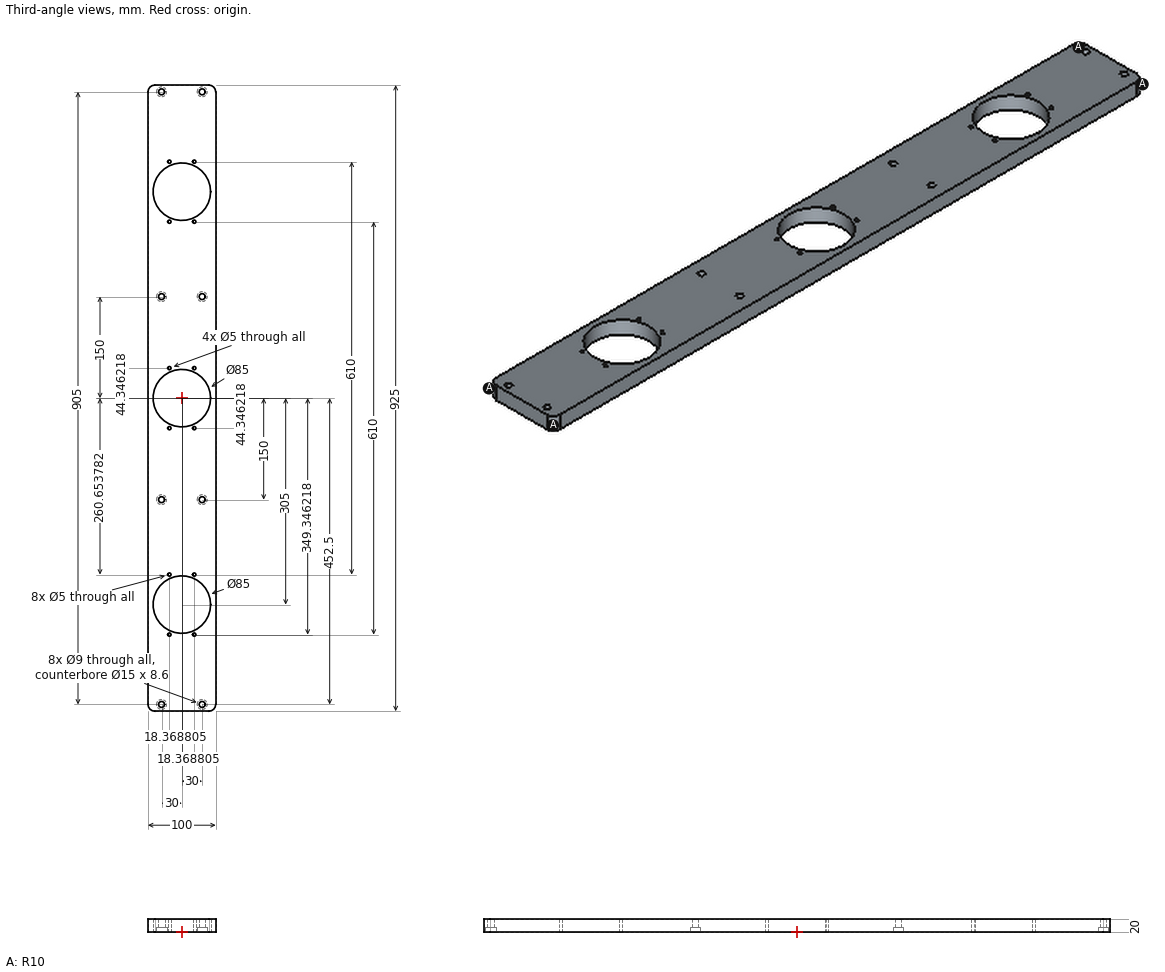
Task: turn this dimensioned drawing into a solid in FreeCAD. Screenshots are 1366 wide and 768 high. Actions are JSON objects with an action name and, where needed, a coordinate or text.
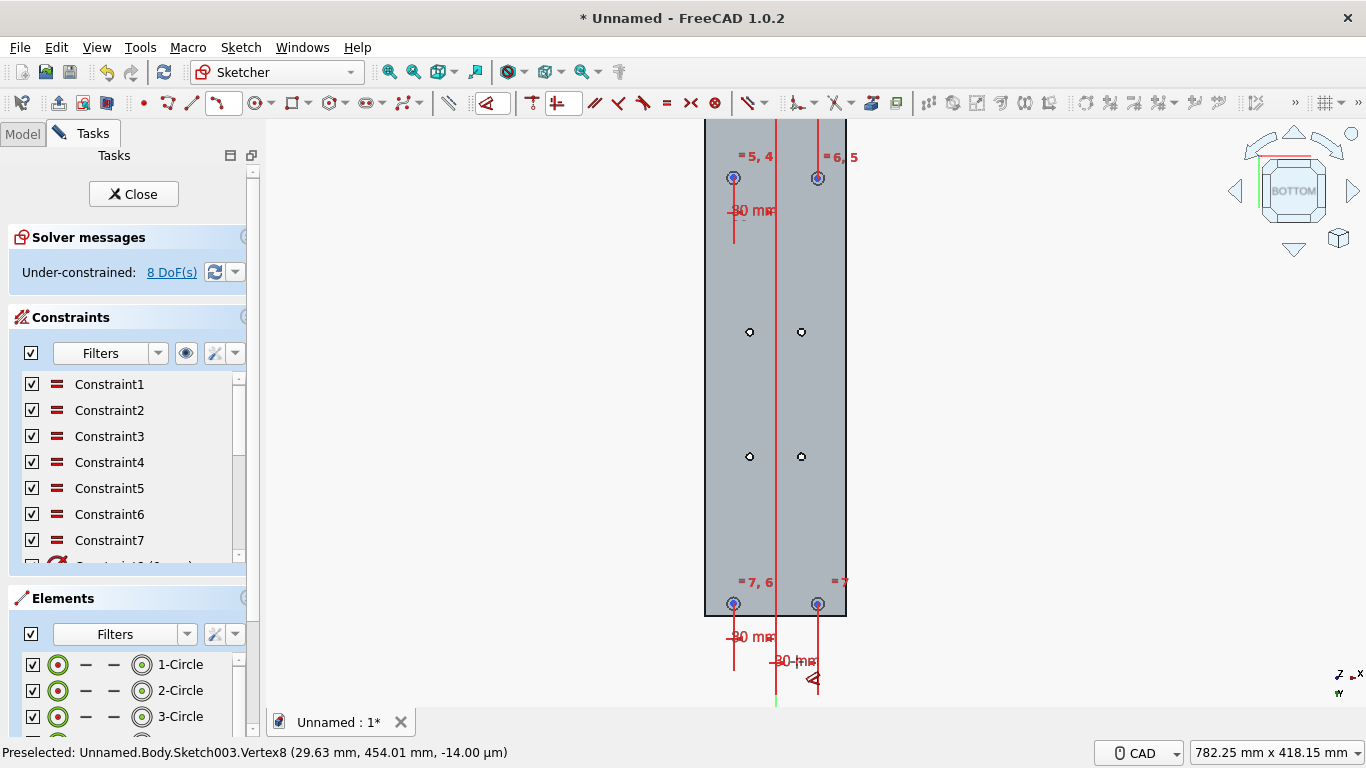
{"action": "scroll", "coordinate": [735, 606], "scroll_direction": "down", "scroll_amount": 6}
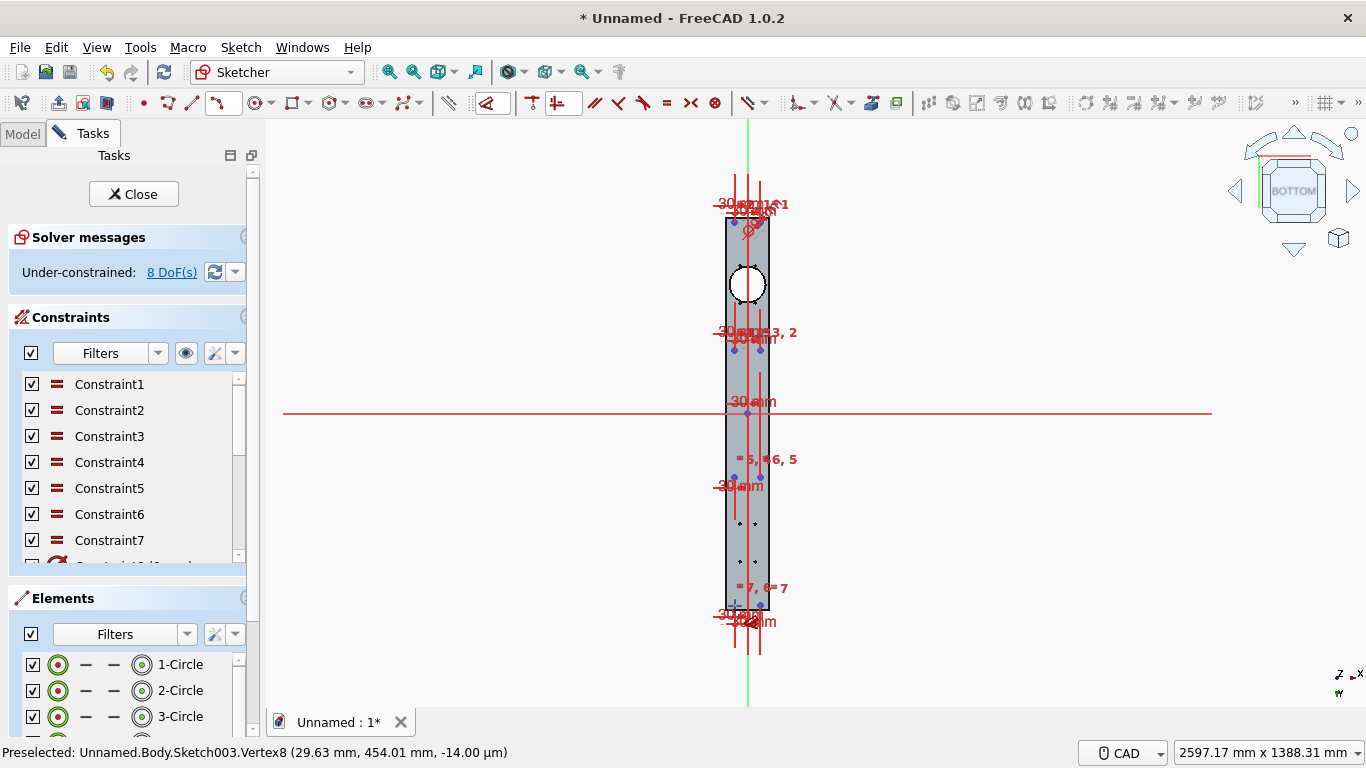
{"action": "left_click", "coordinate": [760, 351]}
{"action": "left_click", "coordinate": [794, 382]}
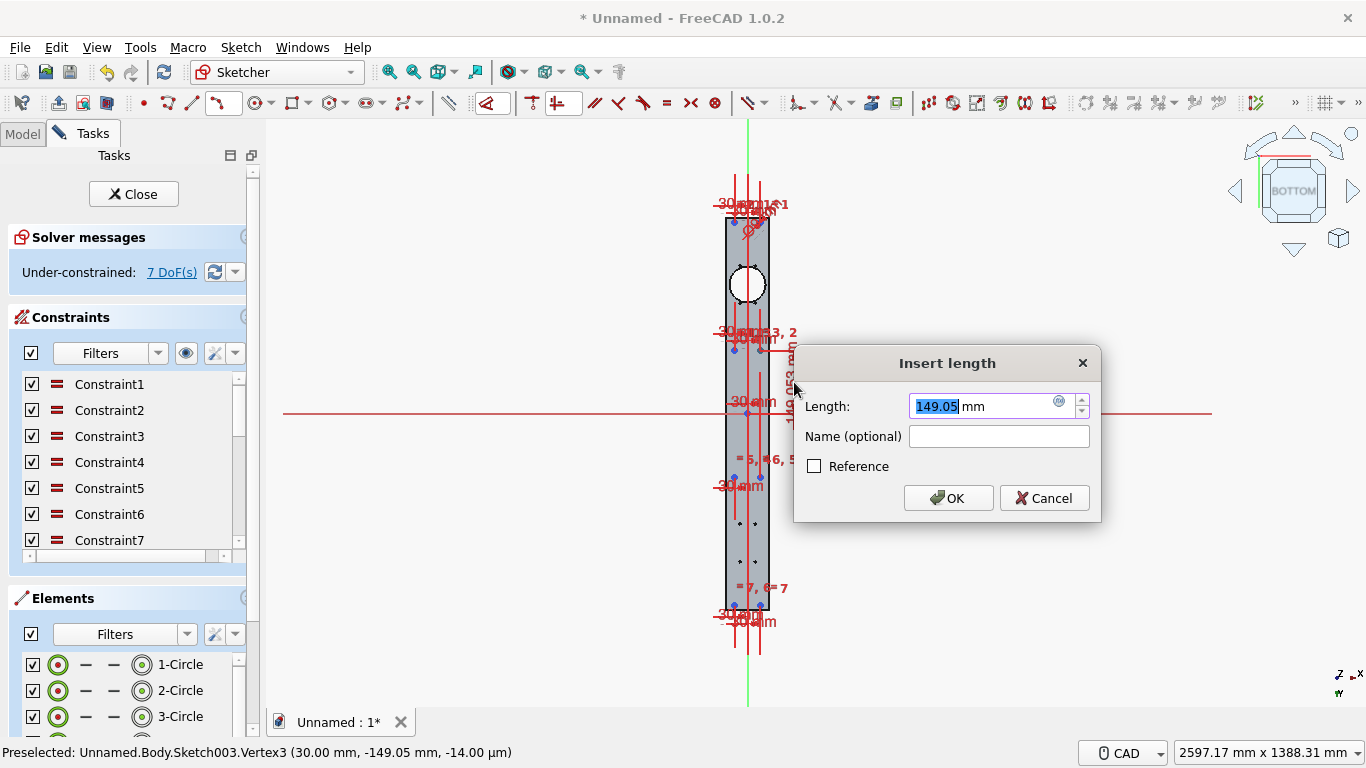
{"action": "type", "text": "150"}
{"action": "key", "text": "Return"}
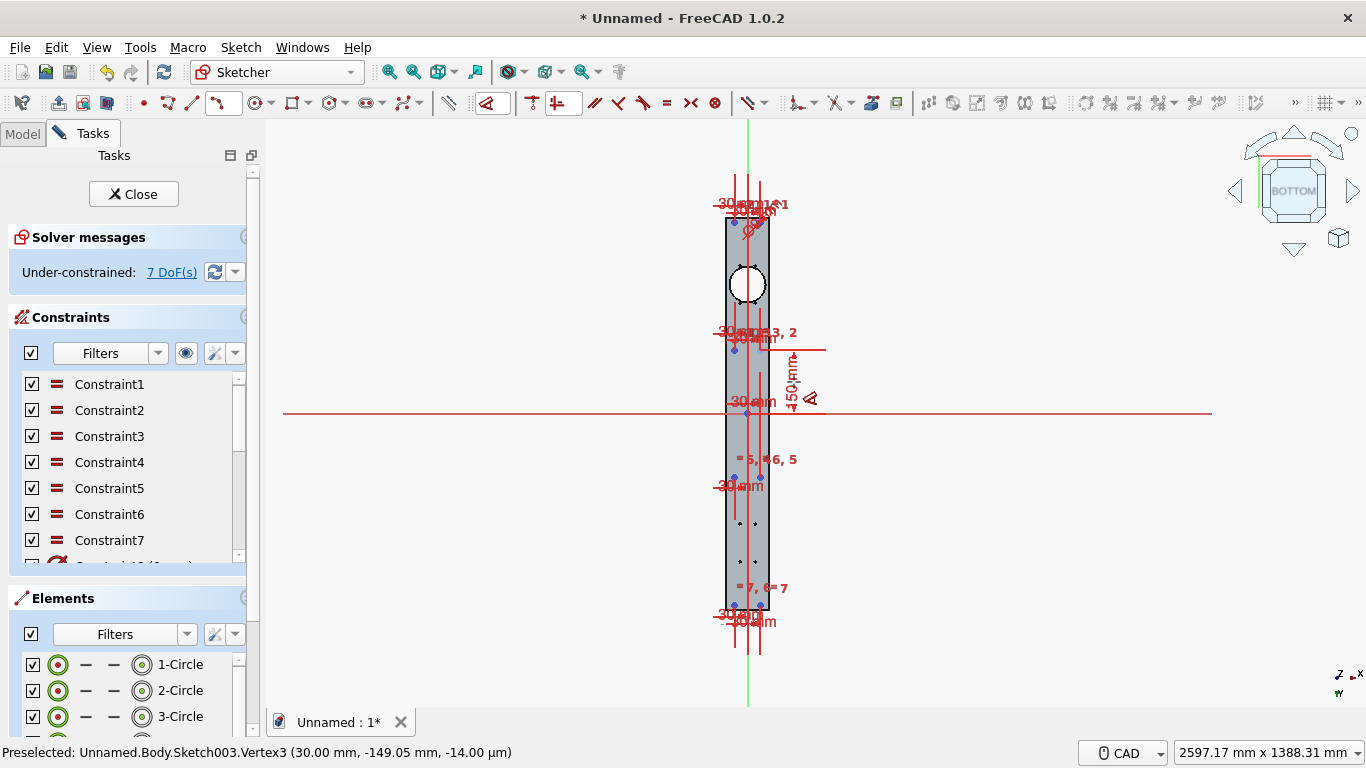
{"action": "left_click", "coordinate": [735, 351]}
{"action": "left_click", "coordinate": [701, 382]}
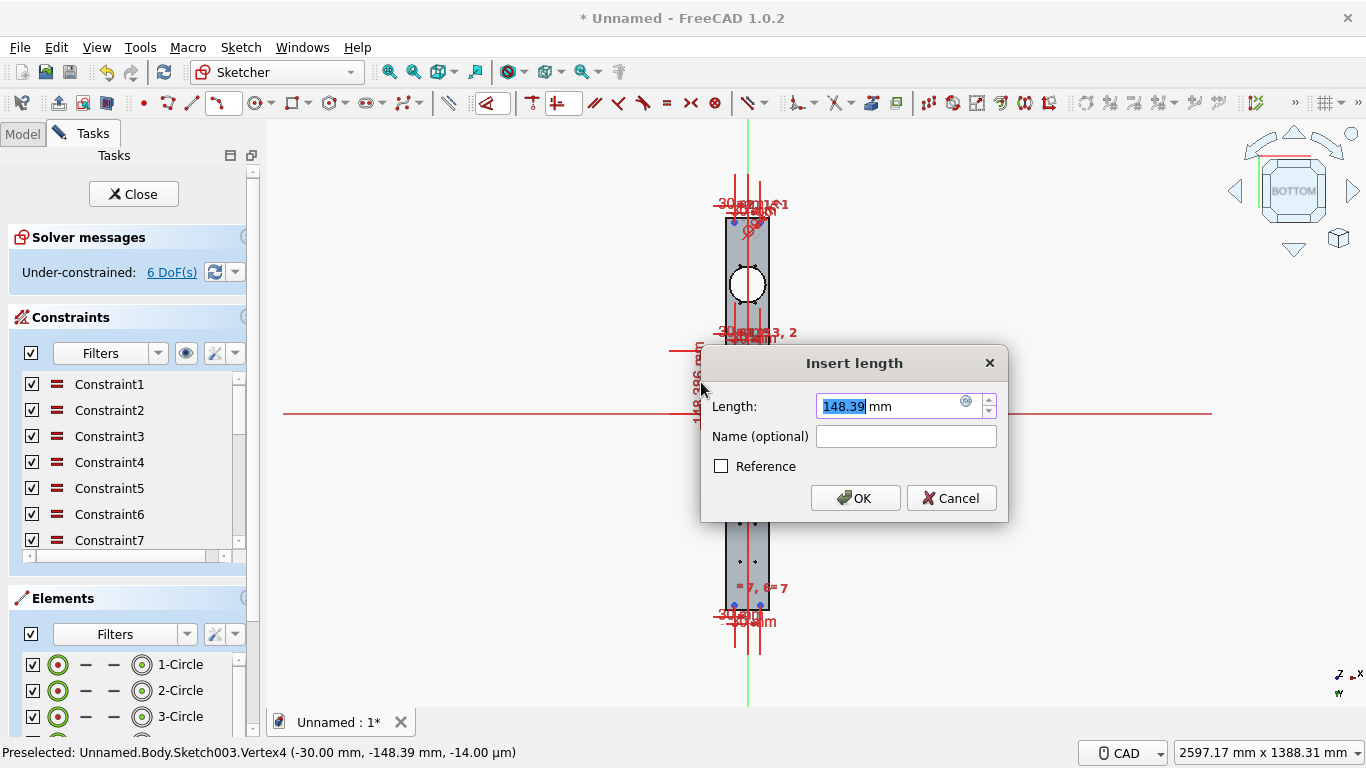
{"action": "type", "text": "150"}
{"action": "key", "text": "Return"}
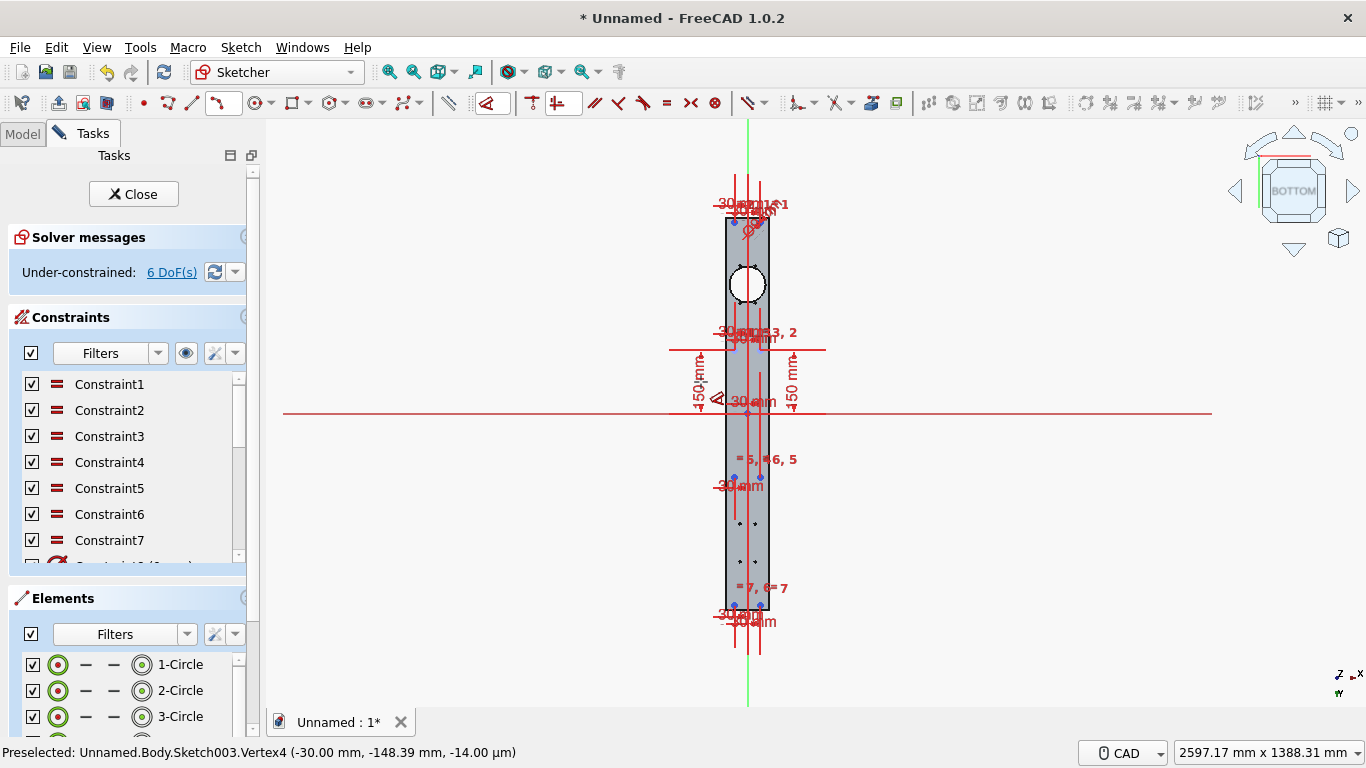
{"action": "left_click", "coordinate": [735, 478]}
{"action": "left_click", "coordinate": [701, 446]}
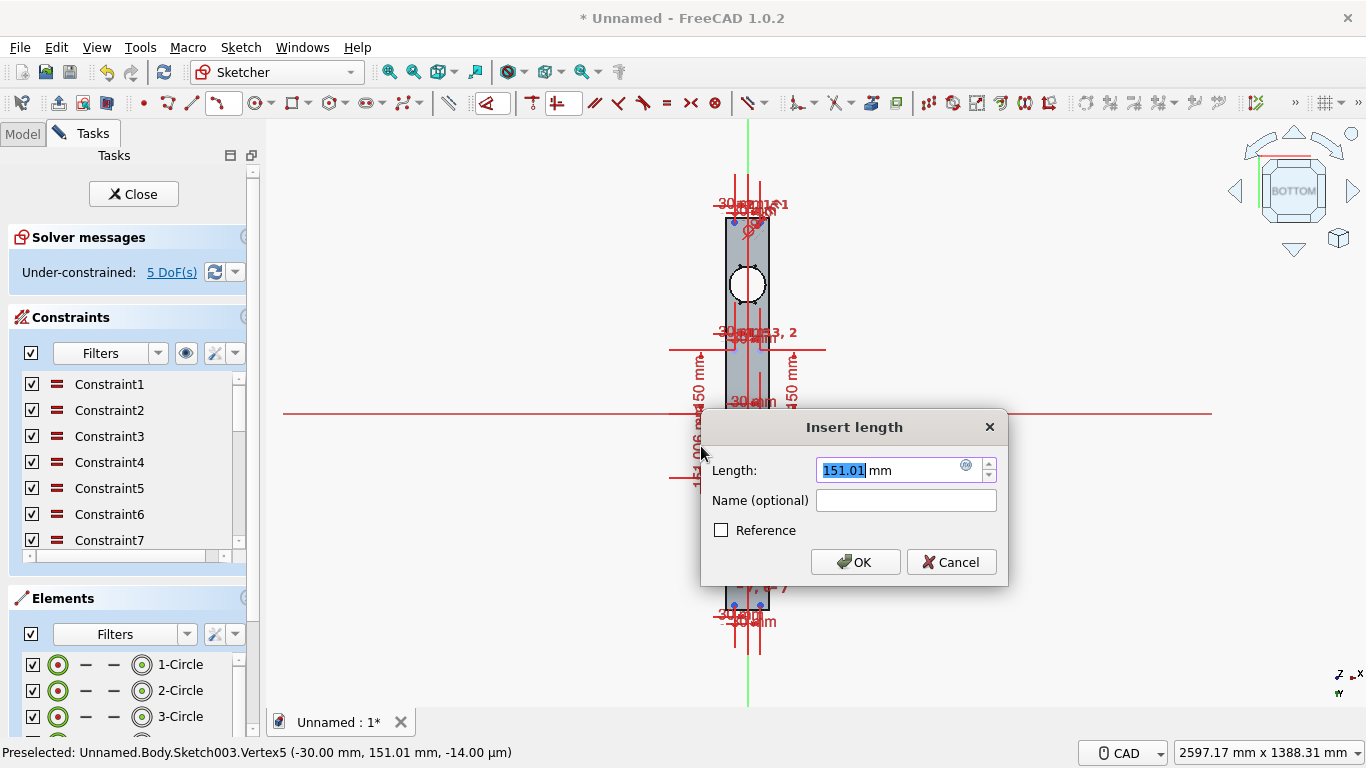
{"action": "type", "text": "150"}
{"action": "key", "text": "Return"}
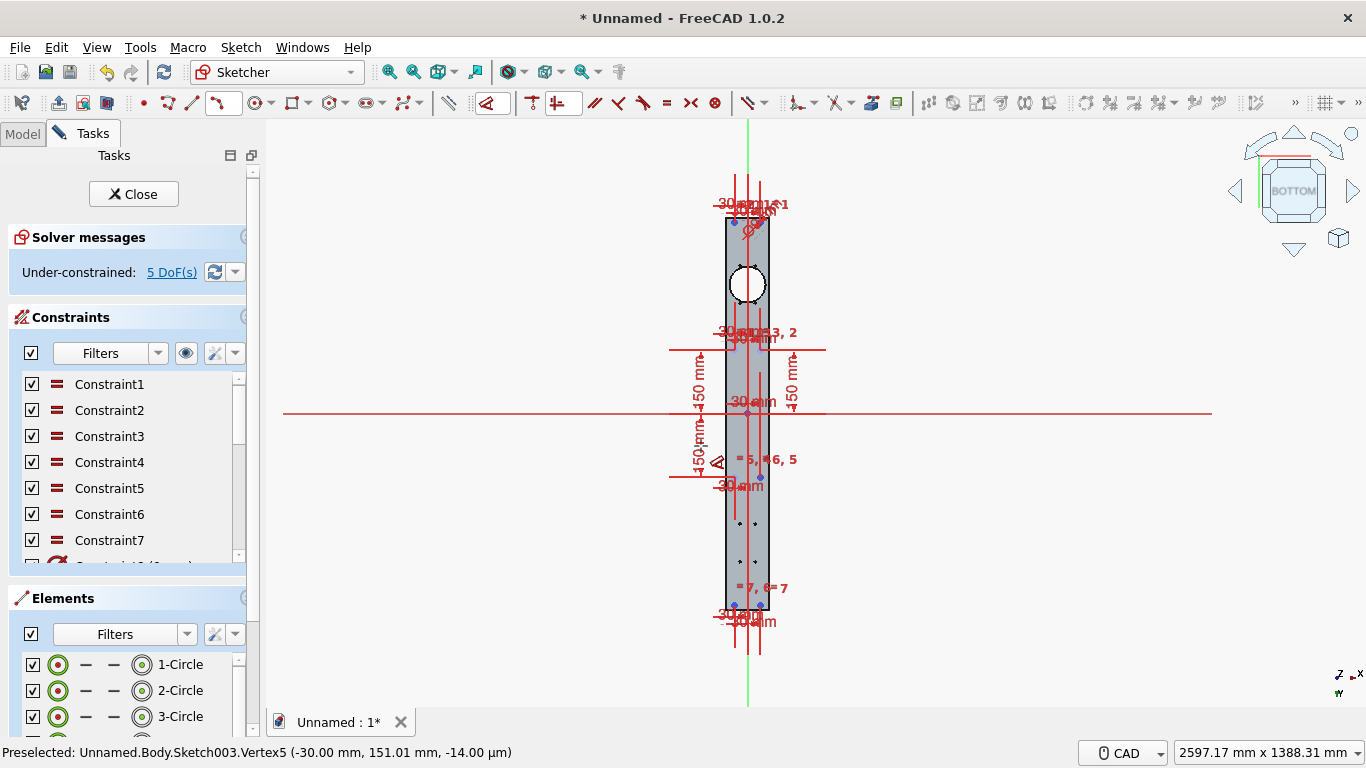
{"action": "left_click", "coordinate": [760, 478]}
{"action": "left_click", "coordinate": [794, 446]}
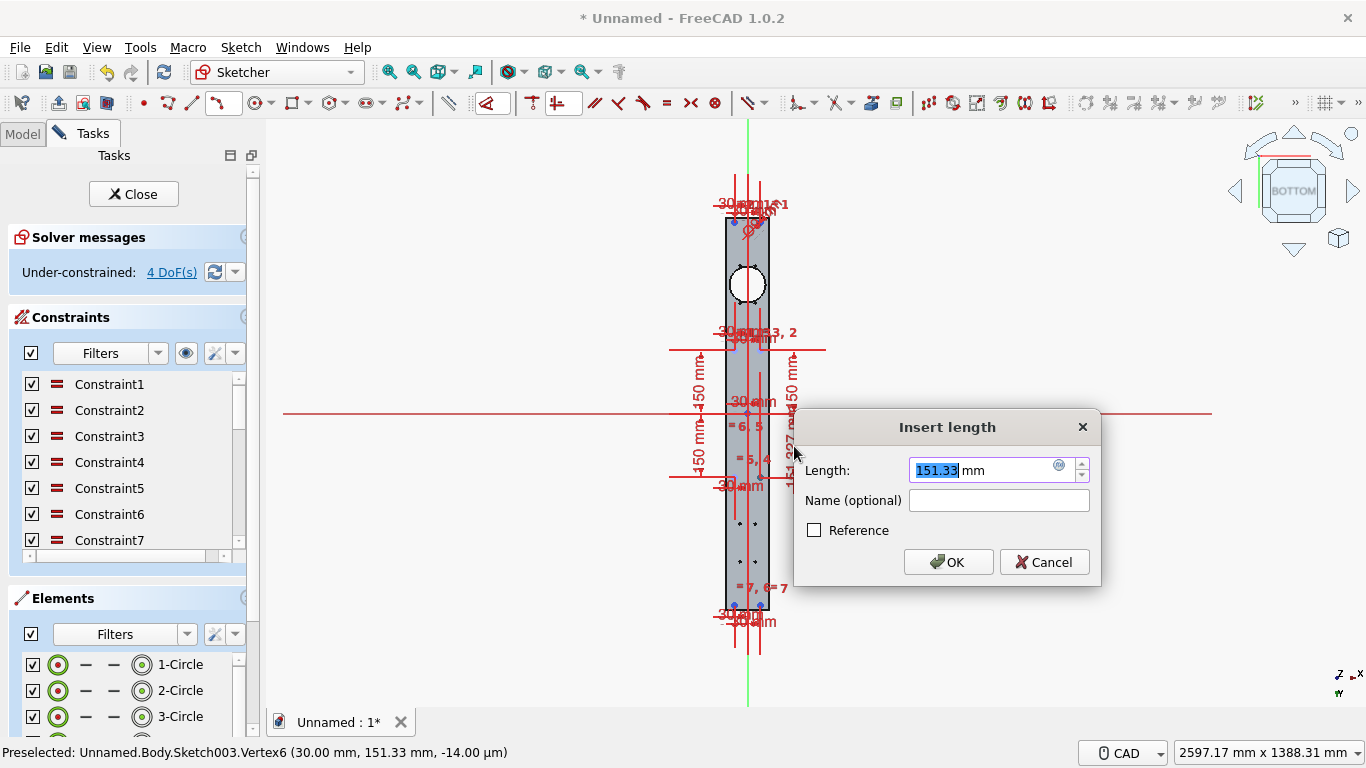
{"action": "type", "text": "150"}
{"action": "key", "text": "Return"}